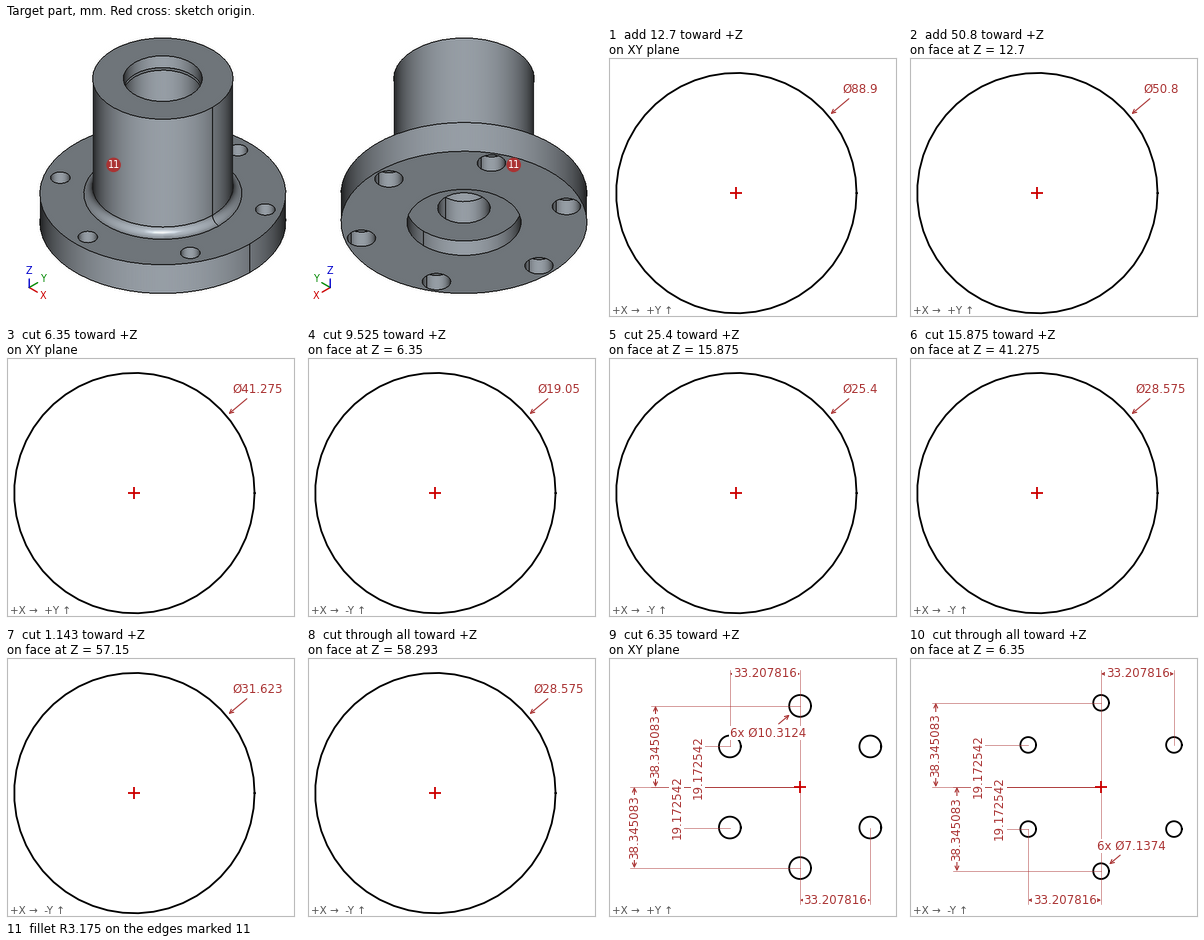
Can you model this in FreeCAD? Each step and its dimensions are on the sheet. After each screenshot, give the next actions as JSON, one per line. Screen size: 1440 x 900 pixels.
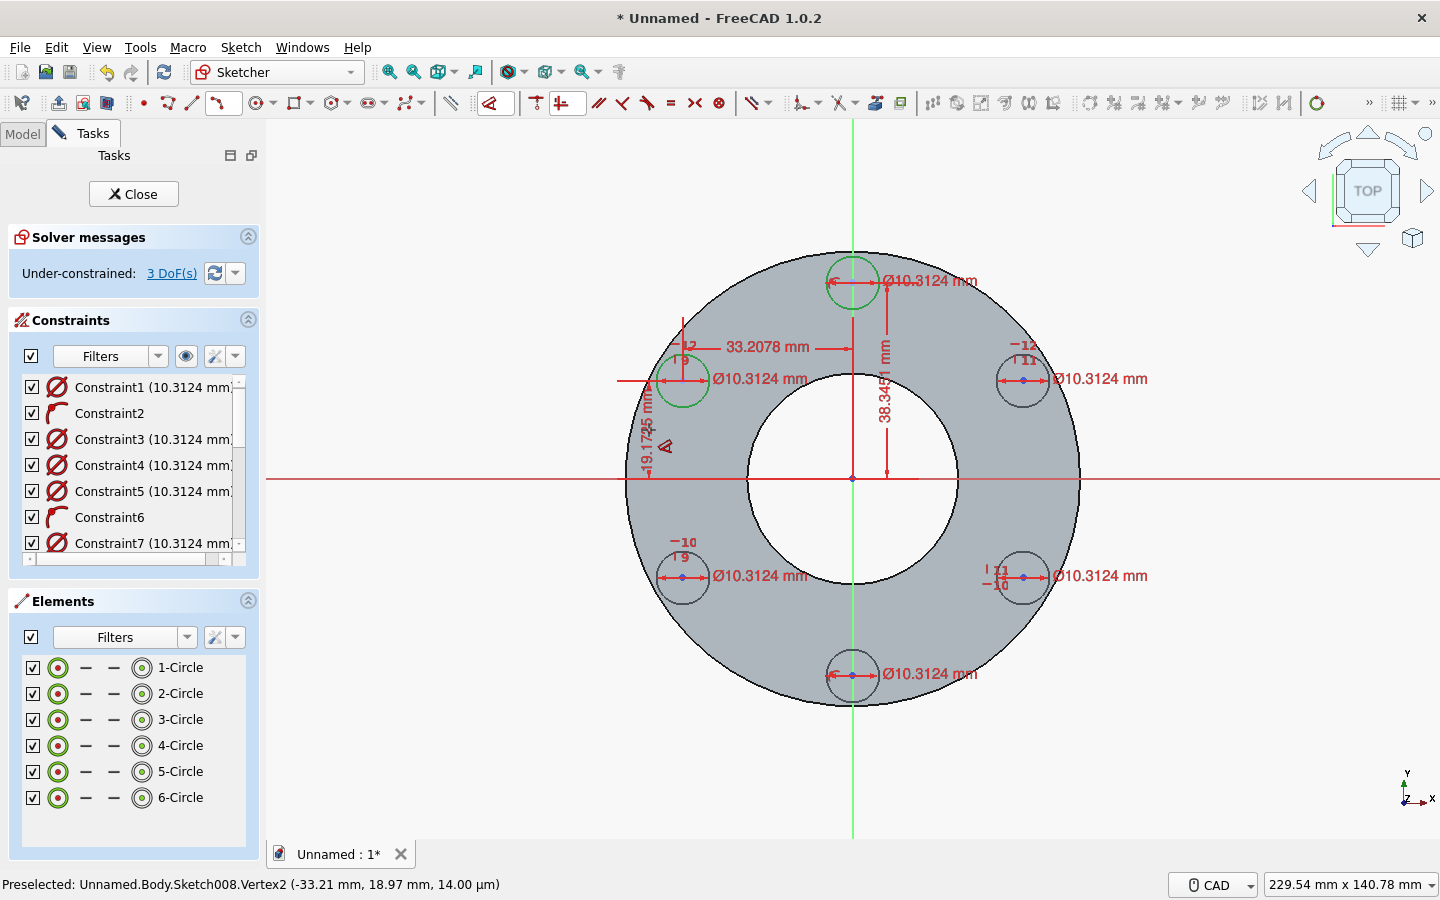
{"action": "left_click", "coordinate": [683, 578]}
{"action": "left_click", "coordinate": [649, 528]}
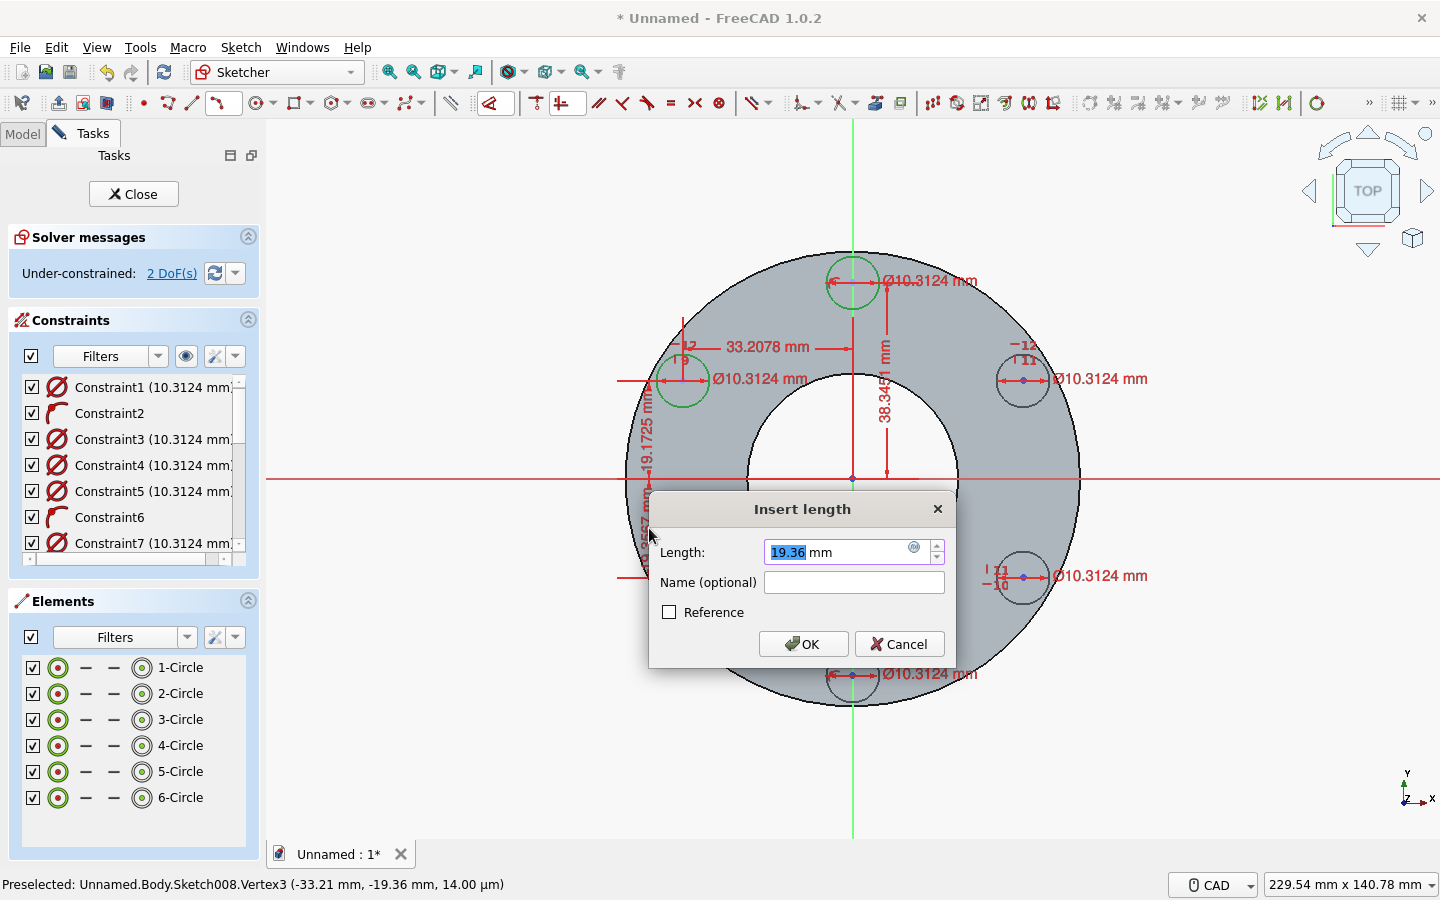
{"action": "type", "text": "19.172542"}
{"action": "key", "text": "Return"}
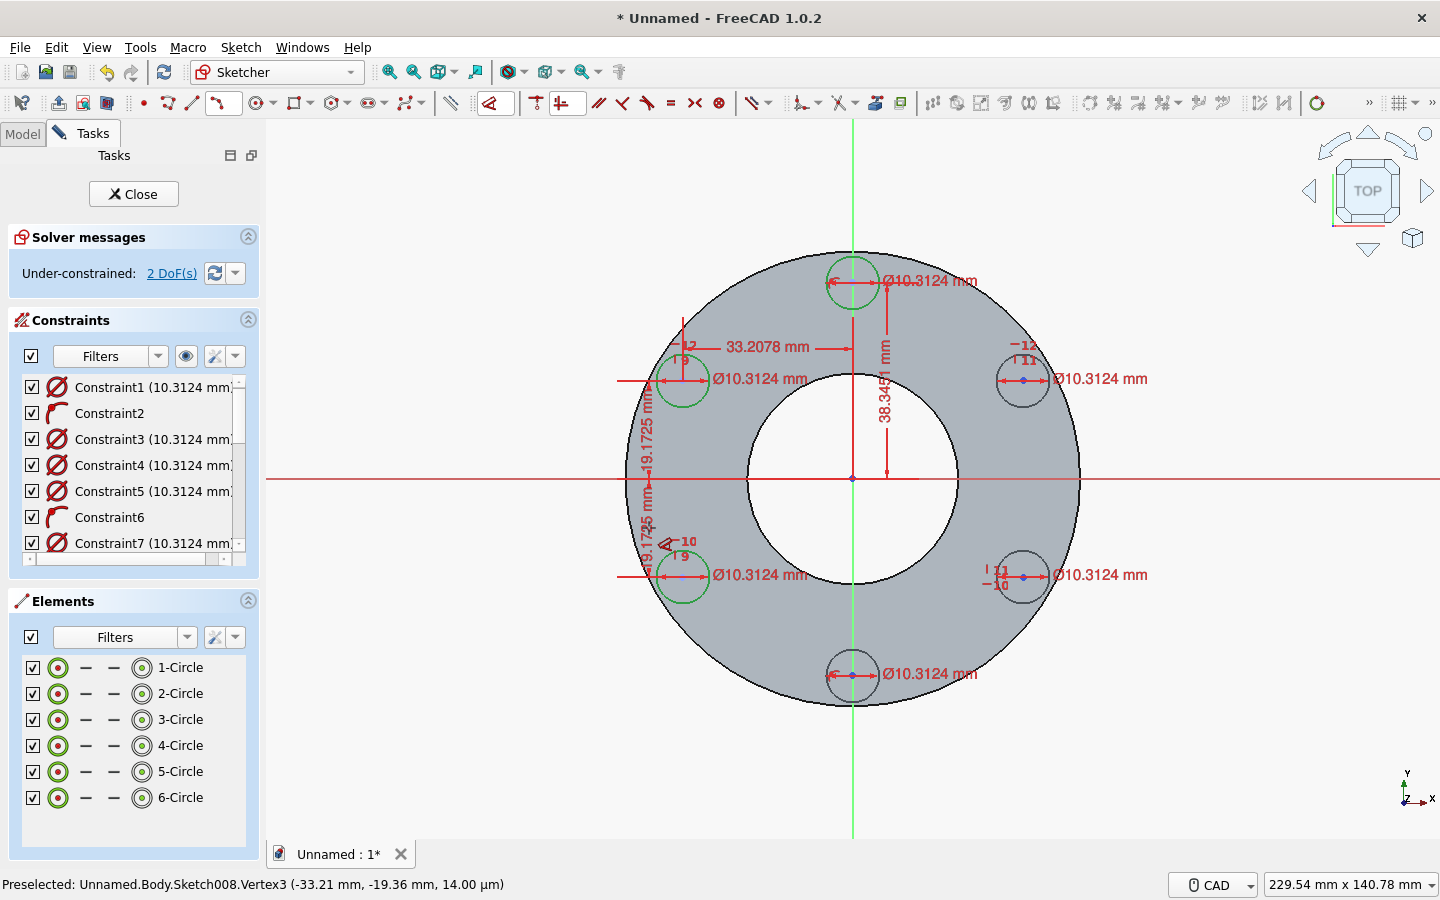
{"action": "left_click", "coordinate": [853, 676]}
{"action": "left_click", "coordinate": [887, 577]}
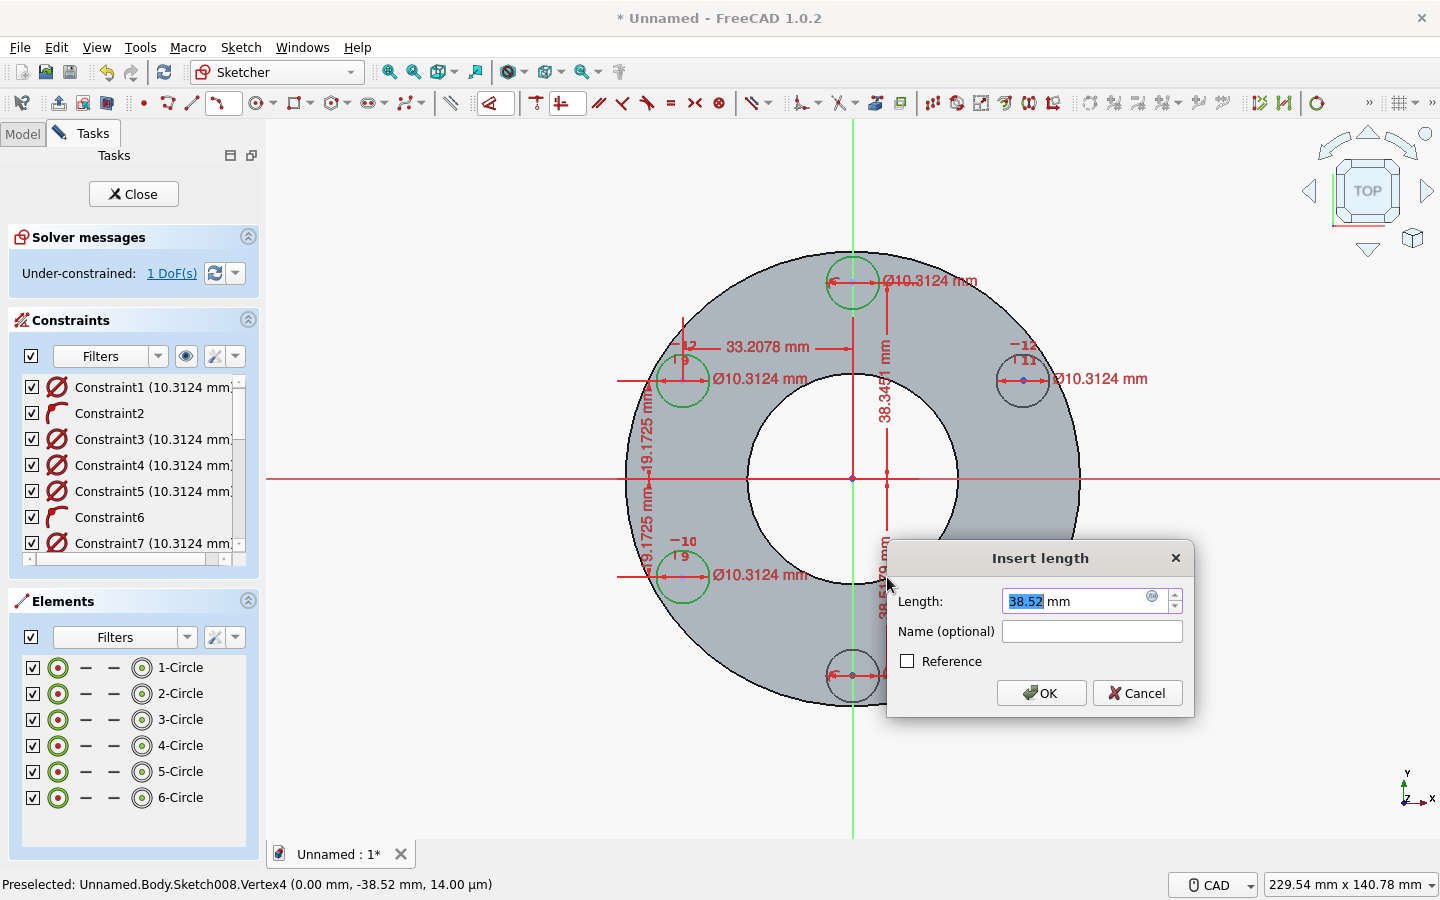
{"action": "type", "text": "38.345083"}
{"action": "key", "text": "Return"}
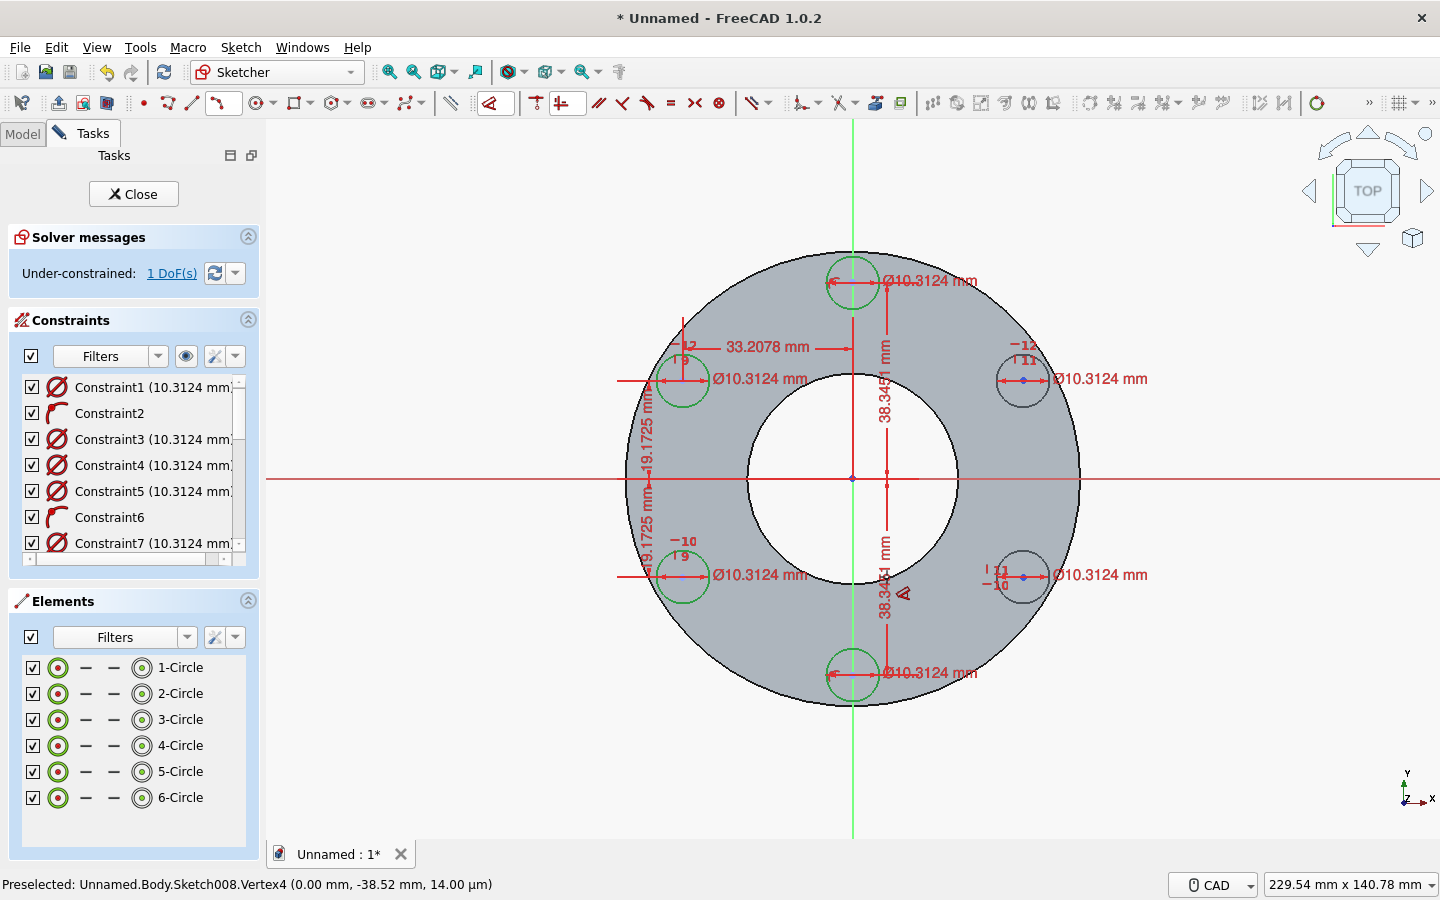
{"action": "left_click", "coordinate": [1023, 577]}
{"action": "left_click", "coordinate": [938, 611]}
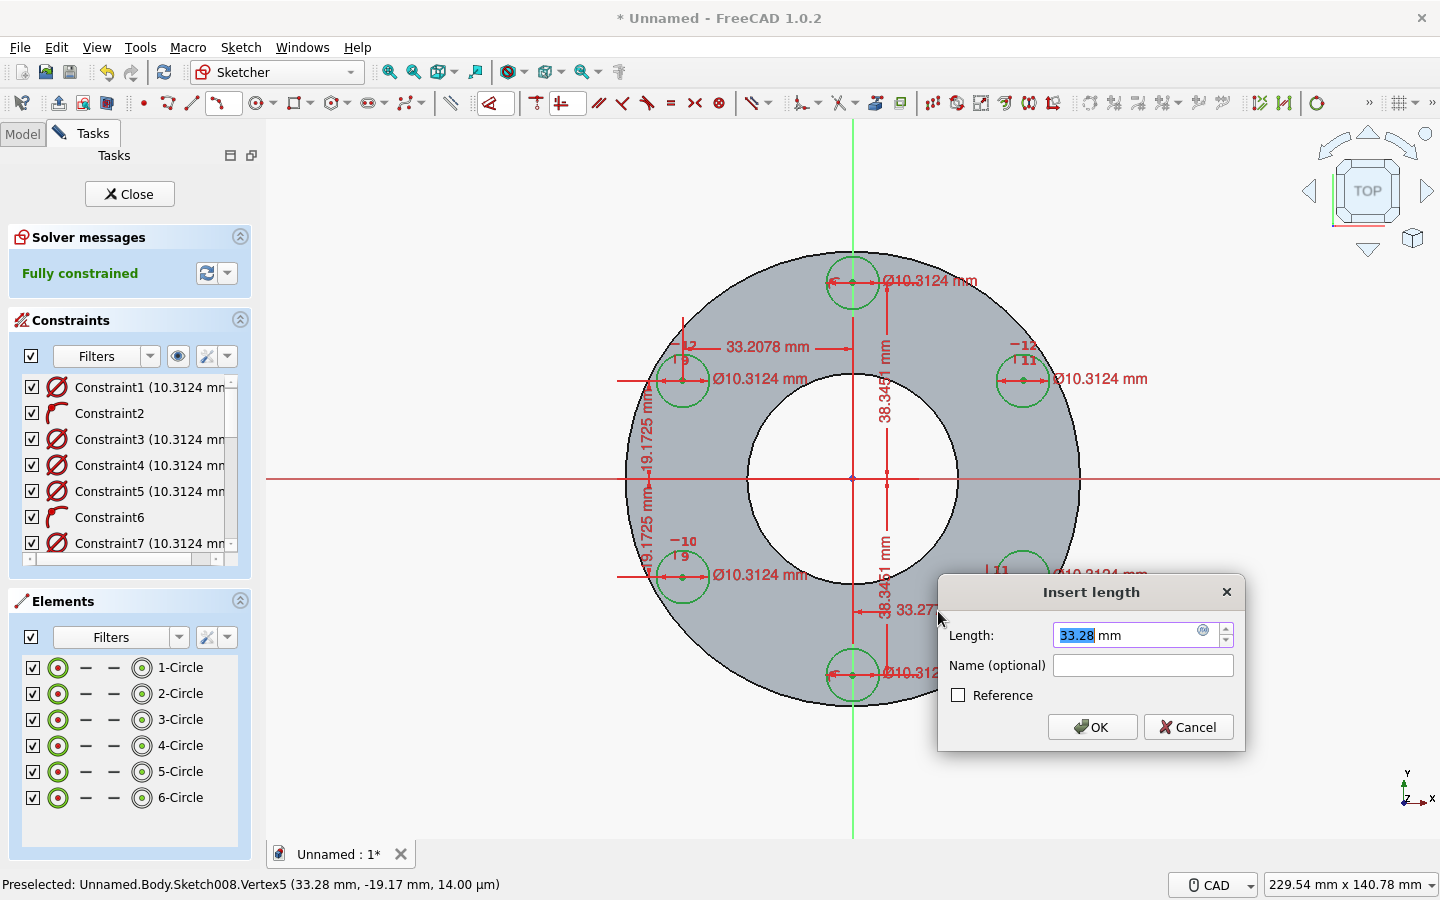
{"action": "type", "text": "33.207816"}
{"action": "key", "text": "Return"}
{"action": "key", "text": "Escape"}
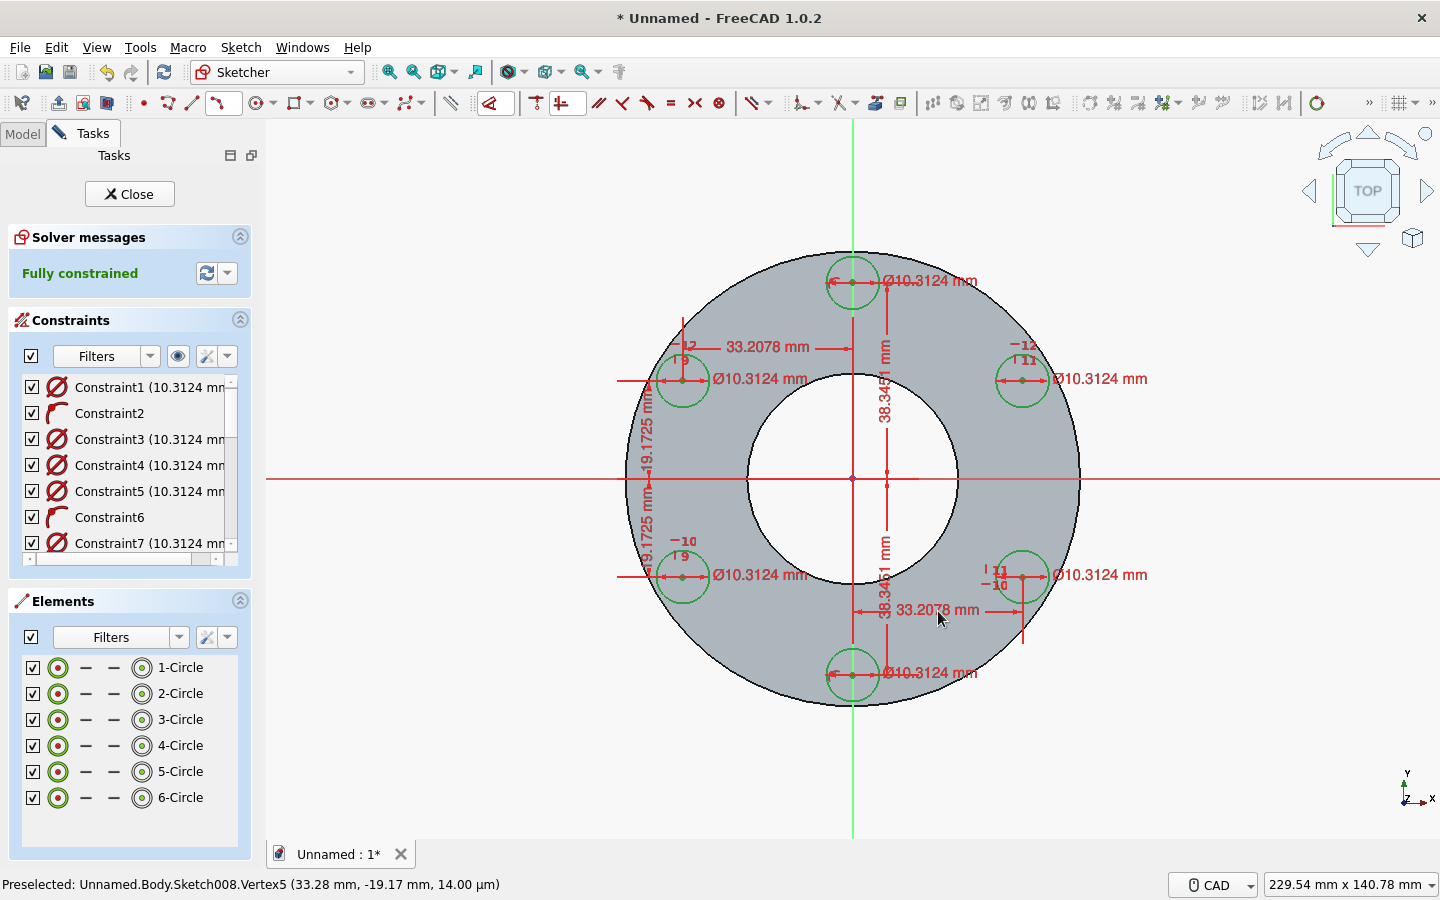
{"action": "left_click", "coordinate": [130, 194]}